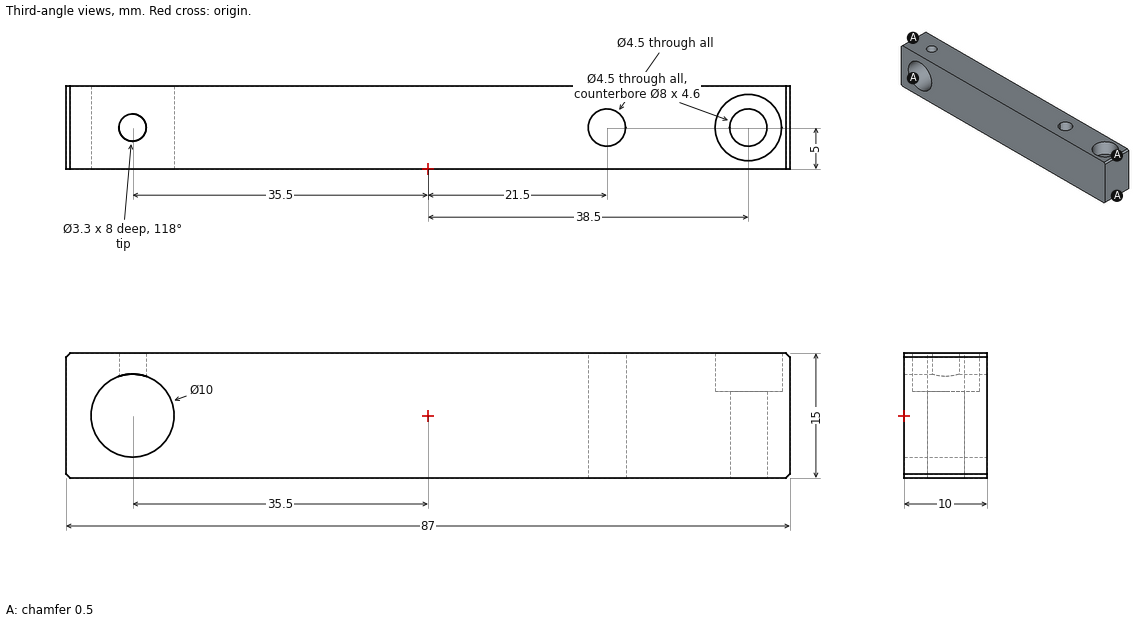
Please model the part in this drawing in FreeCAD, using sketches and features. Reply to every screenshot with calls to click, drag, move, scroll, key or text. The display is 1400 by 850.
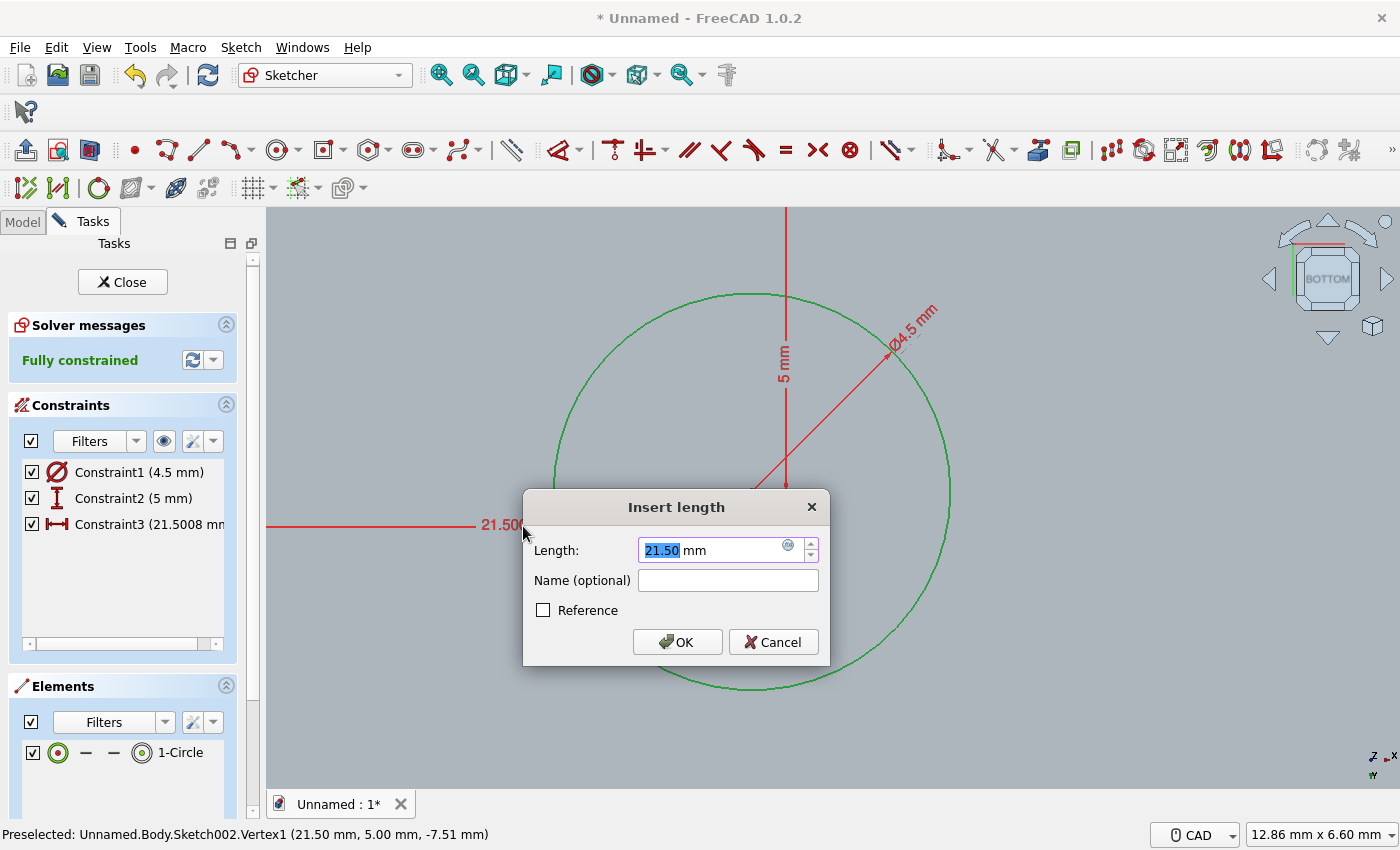
text(21.5)
key(Return)
key(Escape)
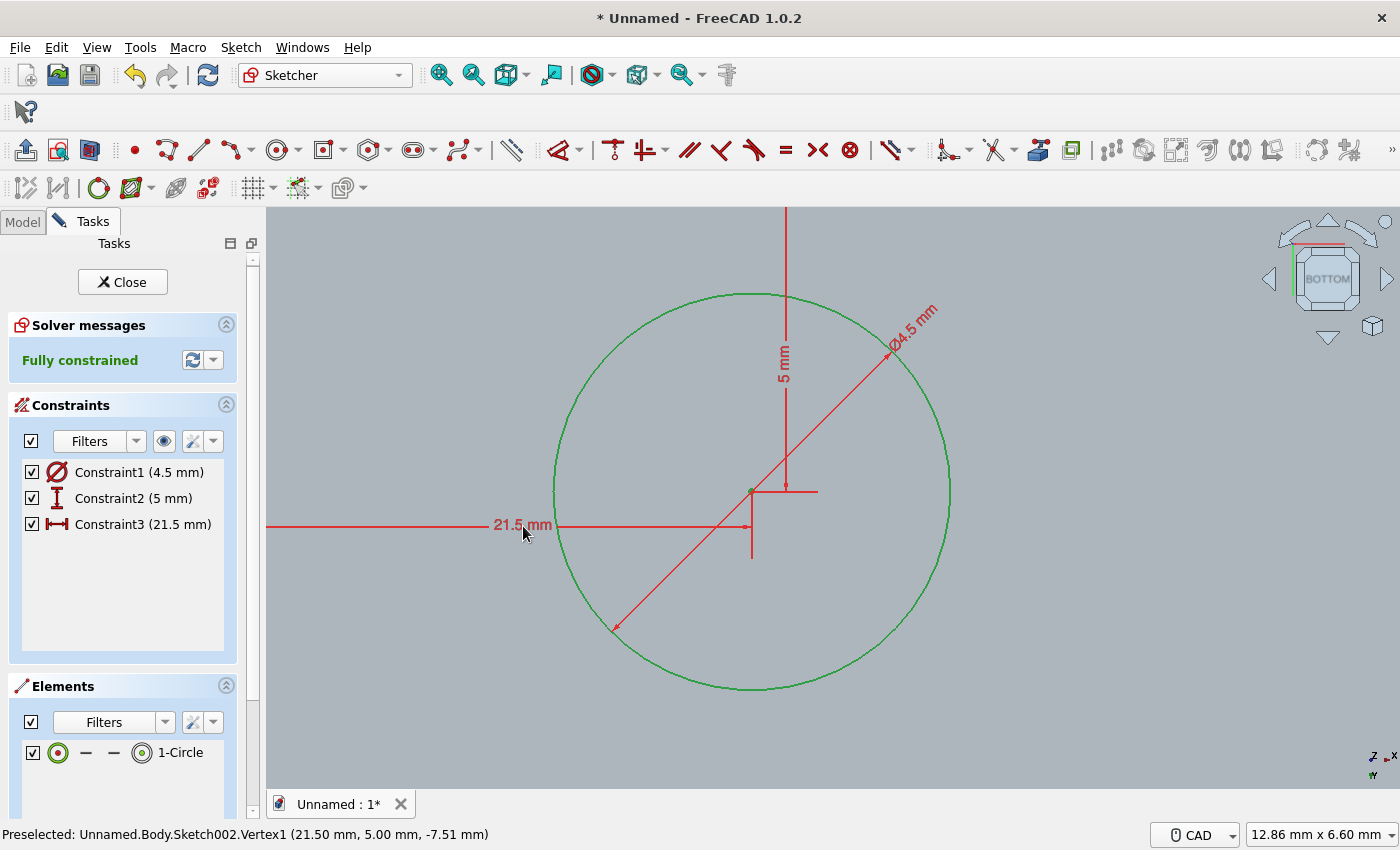
click(123, 282)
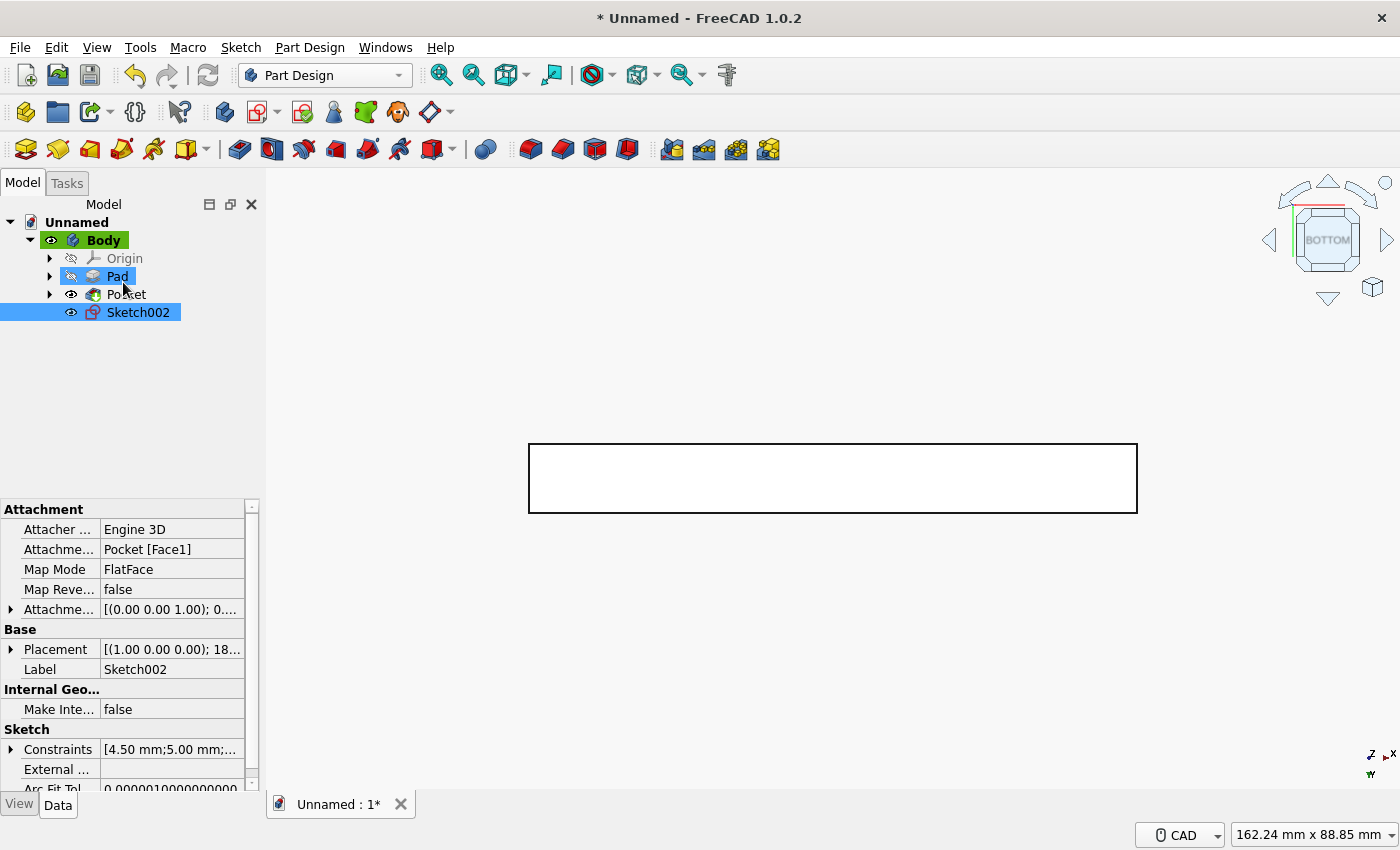
click(272, 150)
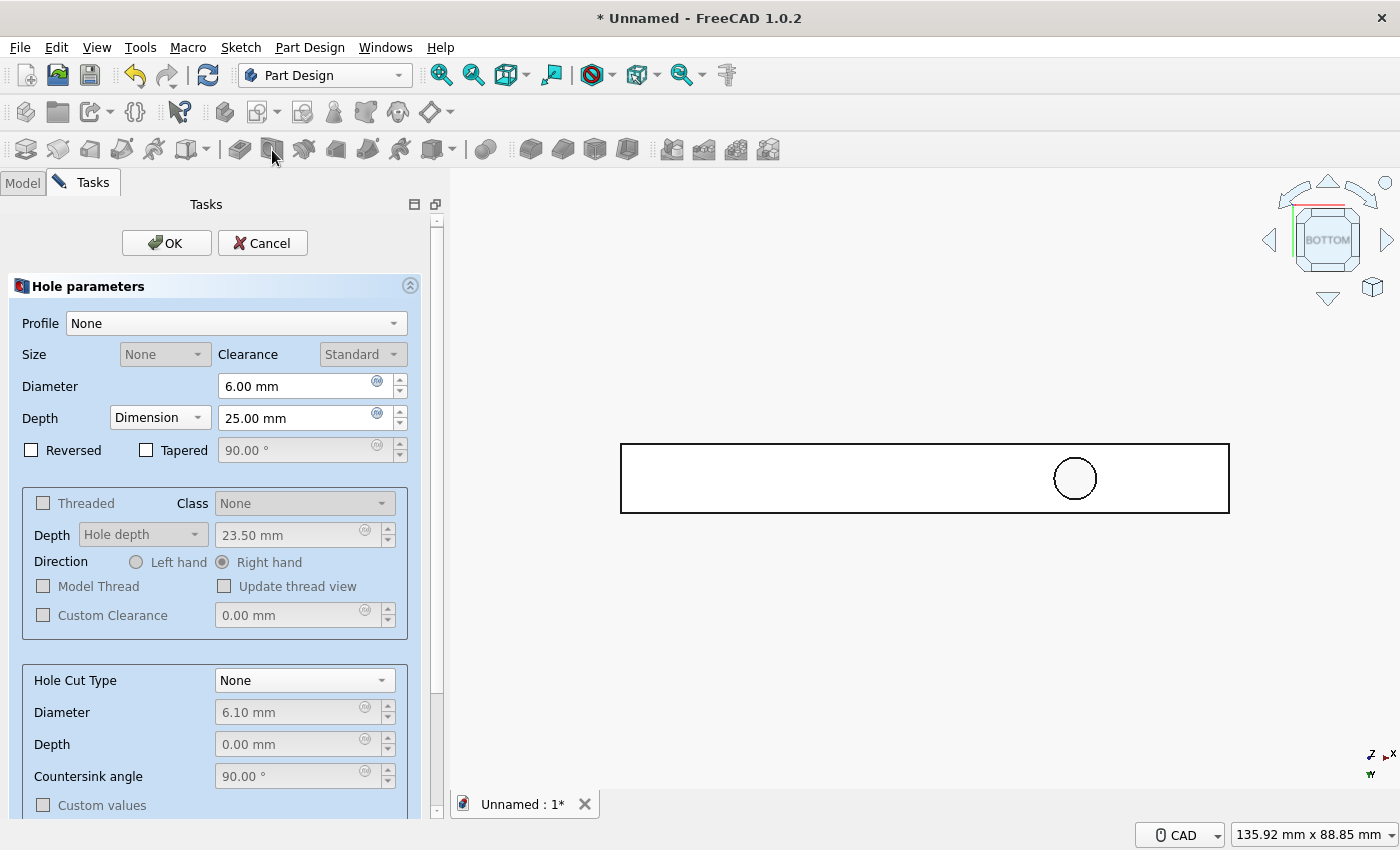
triple_click(305, 386)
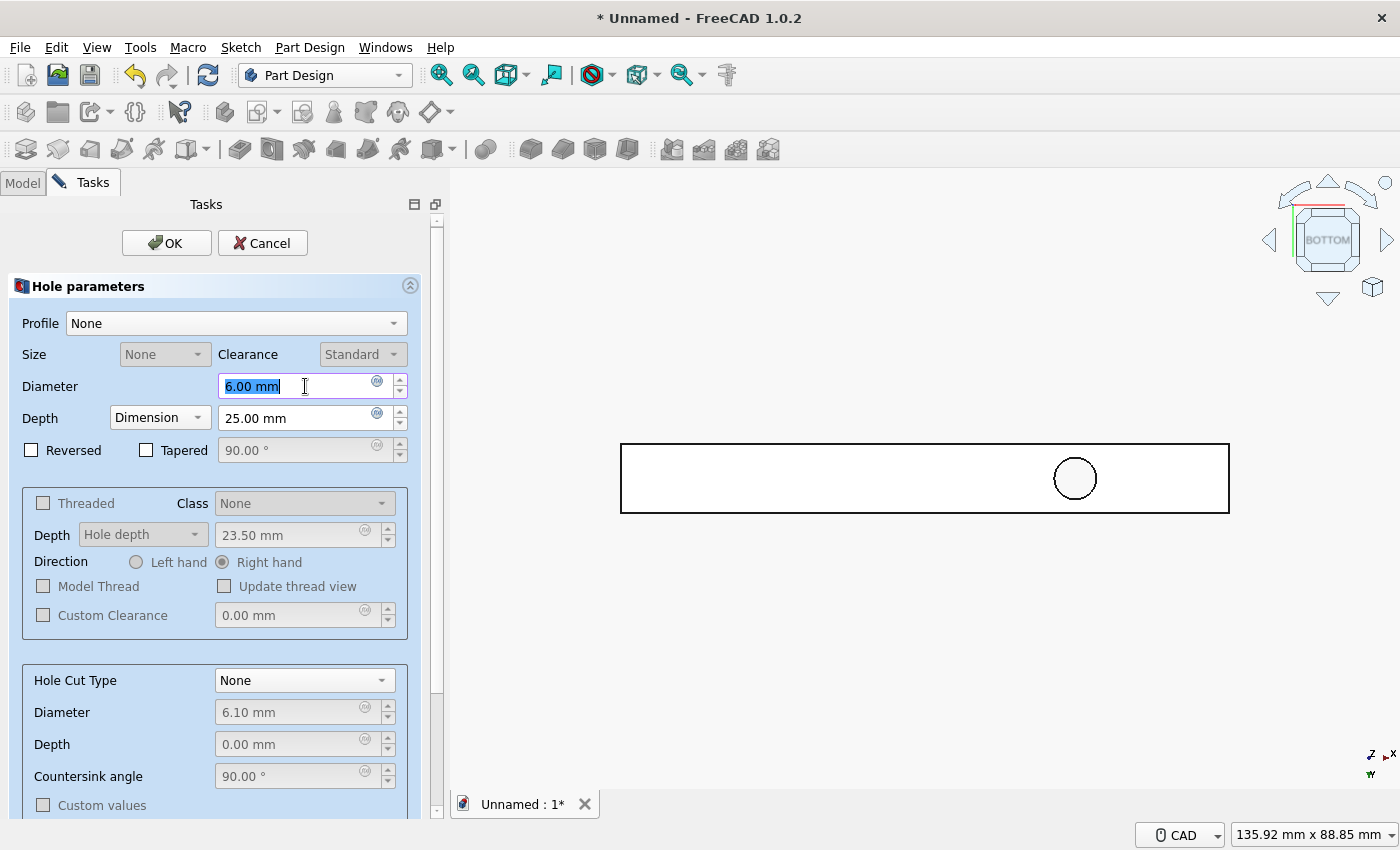
text(4.5)
key(Tab)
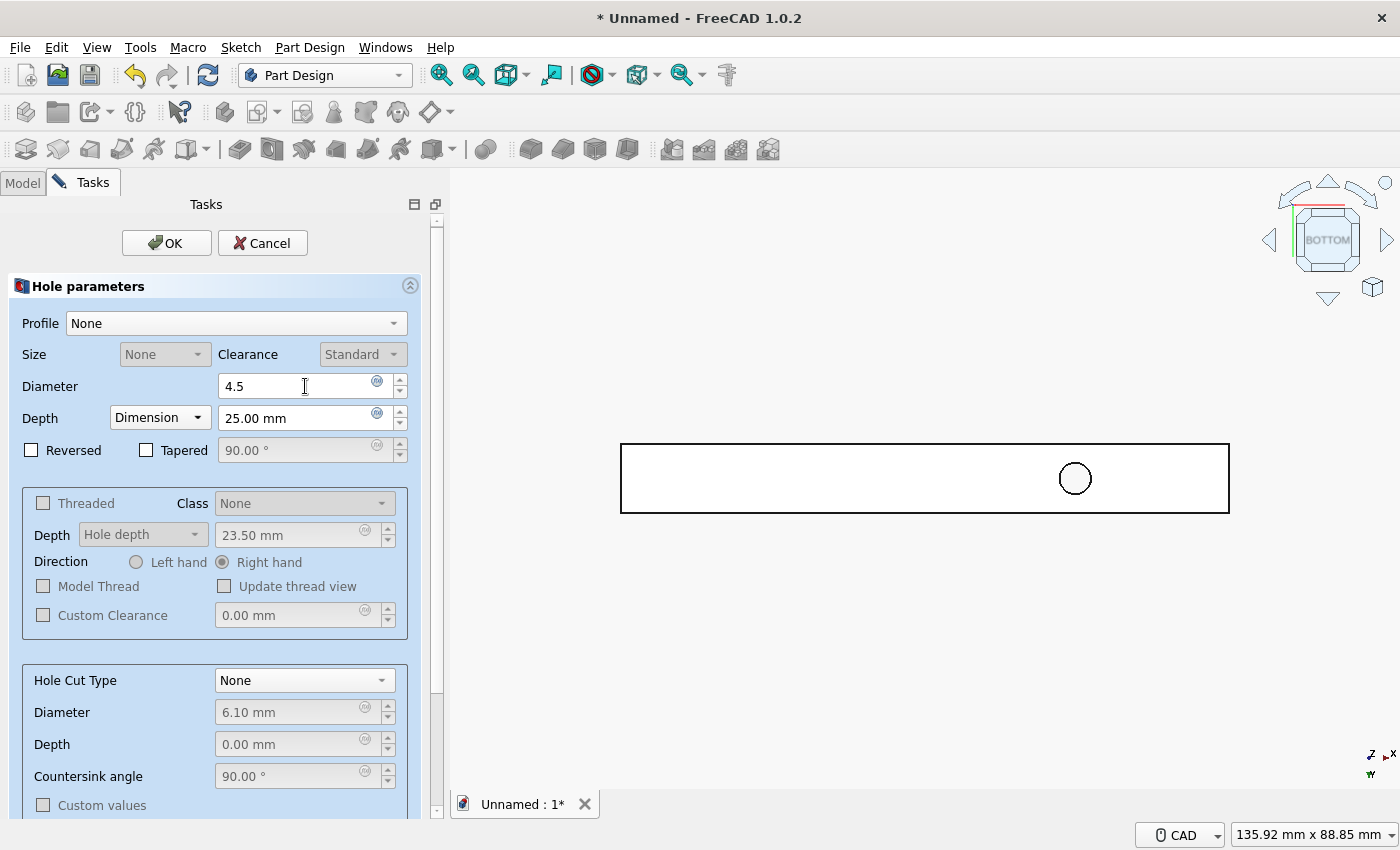
click(161, 418)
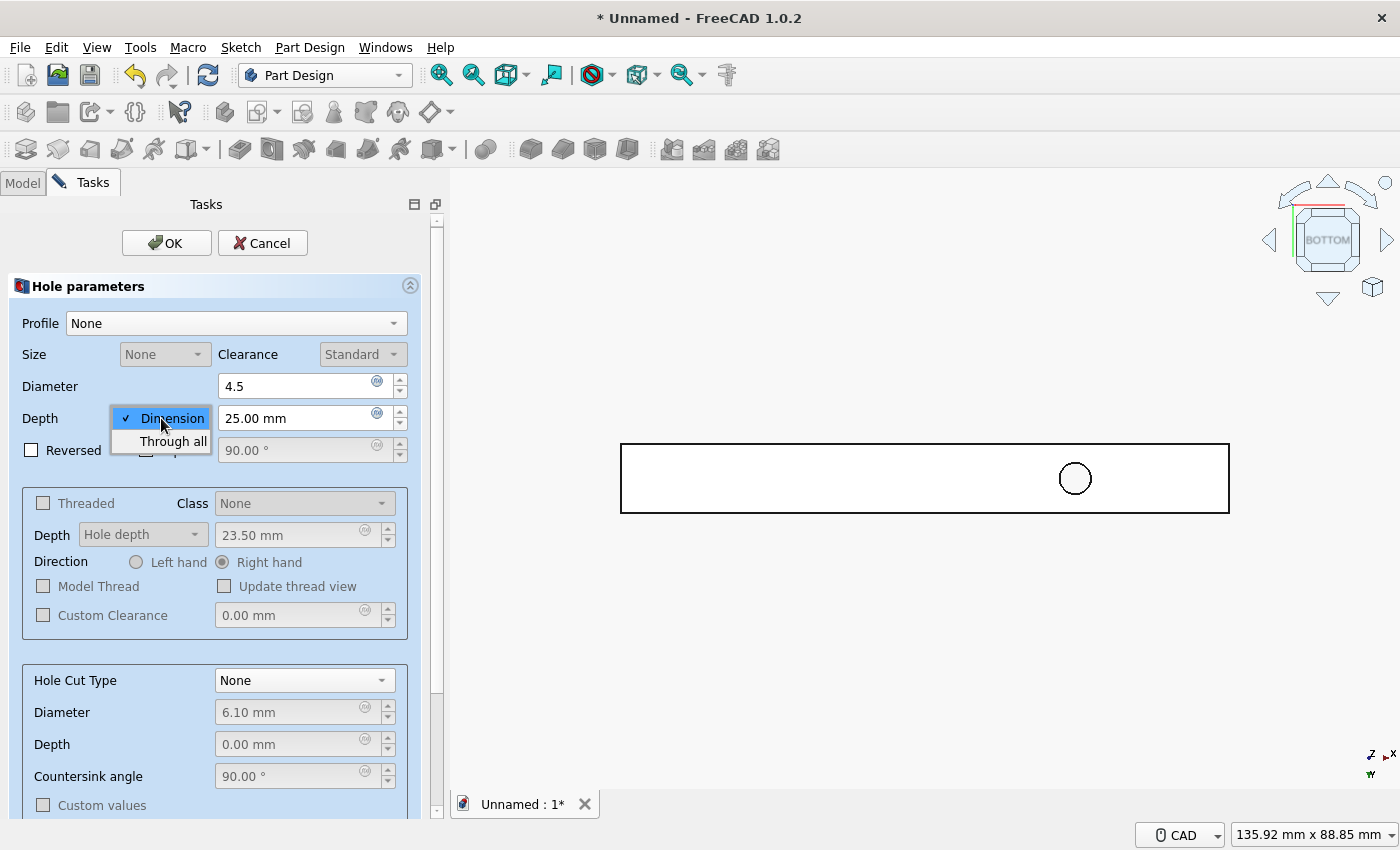
click(160, 442)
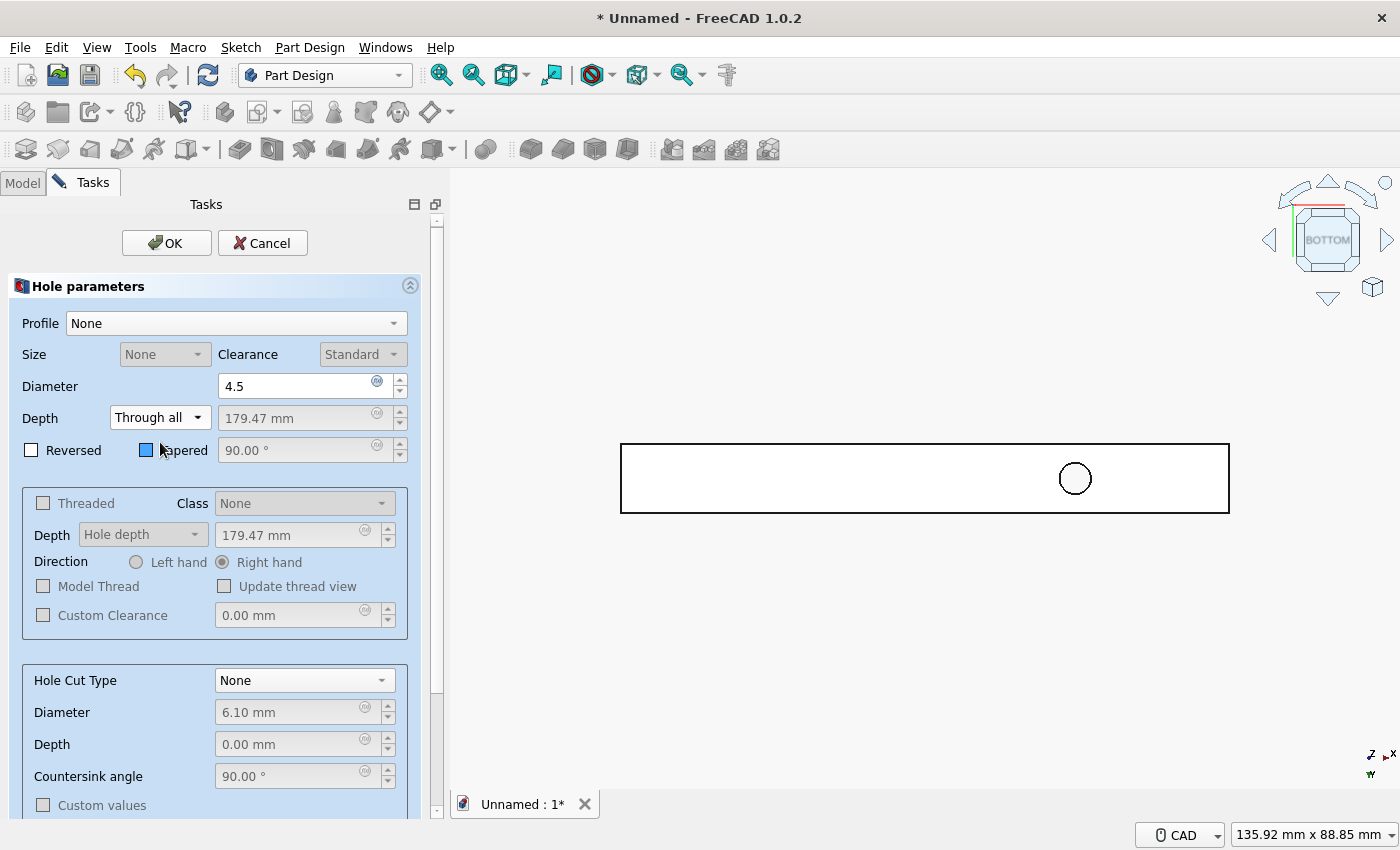
click(167, 243)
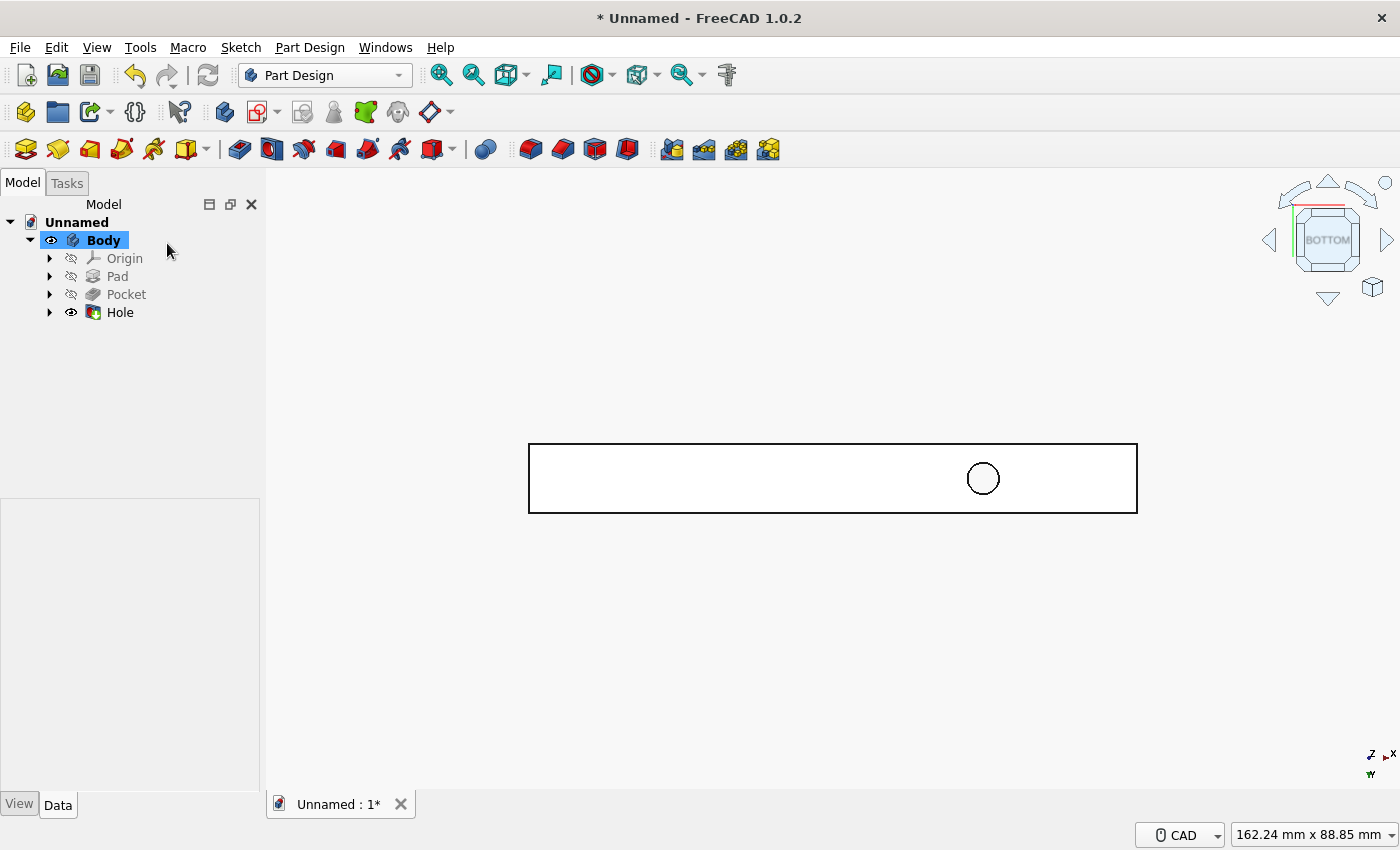
key(0)